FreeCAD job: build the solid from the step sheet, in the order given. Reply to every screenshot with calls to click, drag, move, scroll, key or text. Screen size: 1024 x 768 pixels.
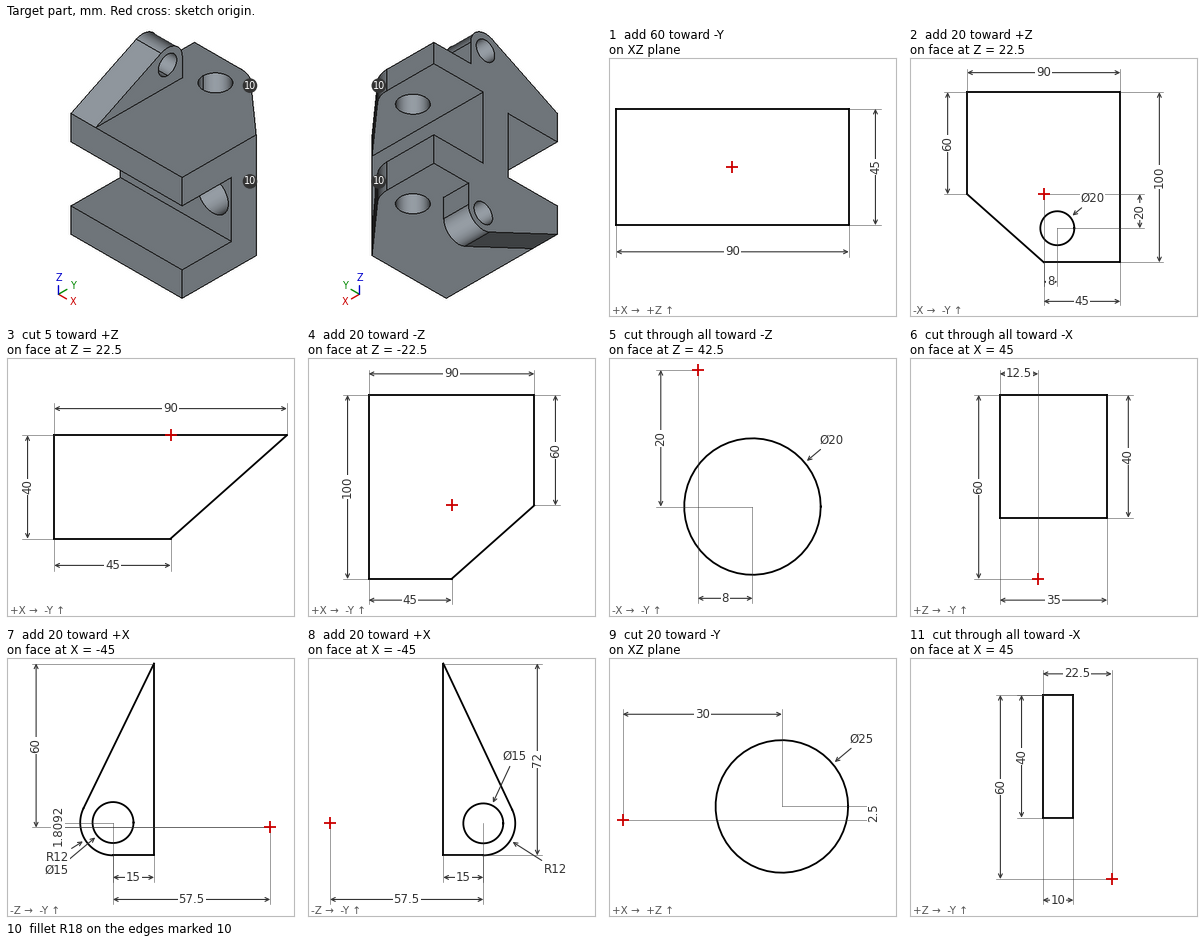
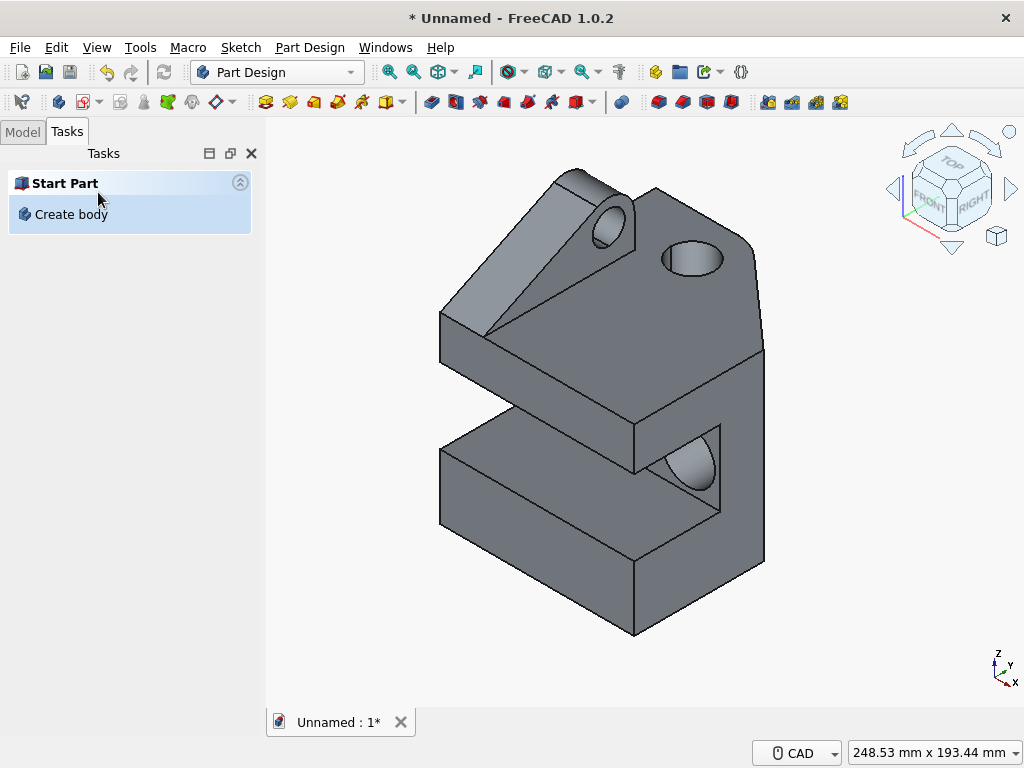
click(736, 531)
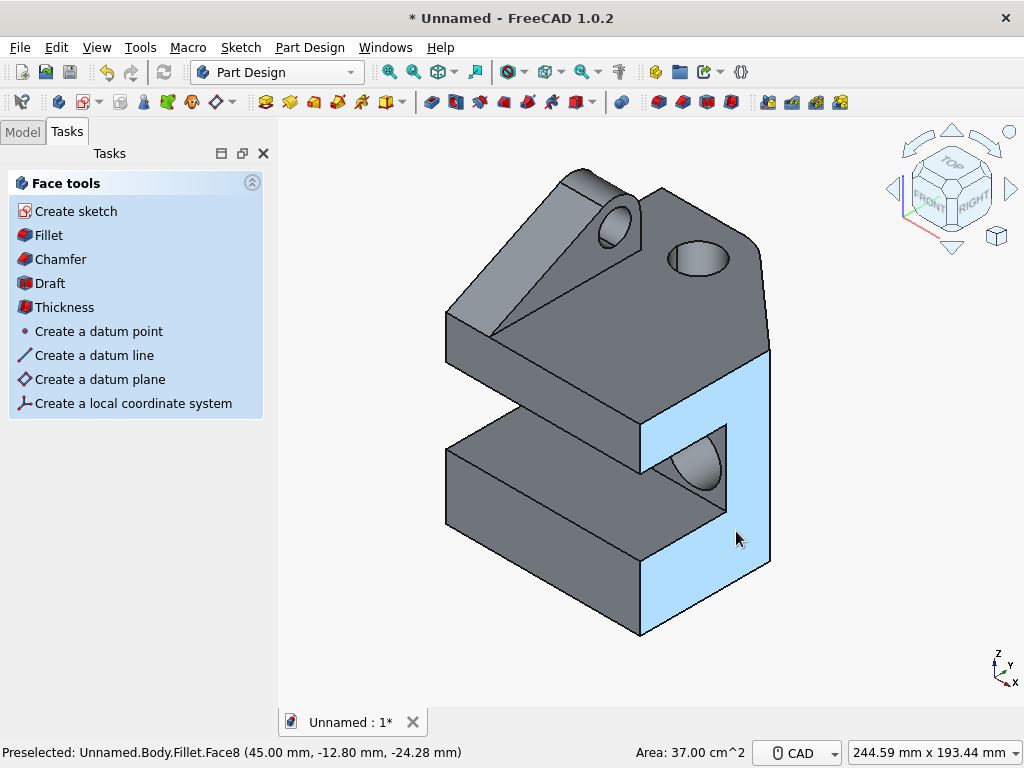
click(84, 102)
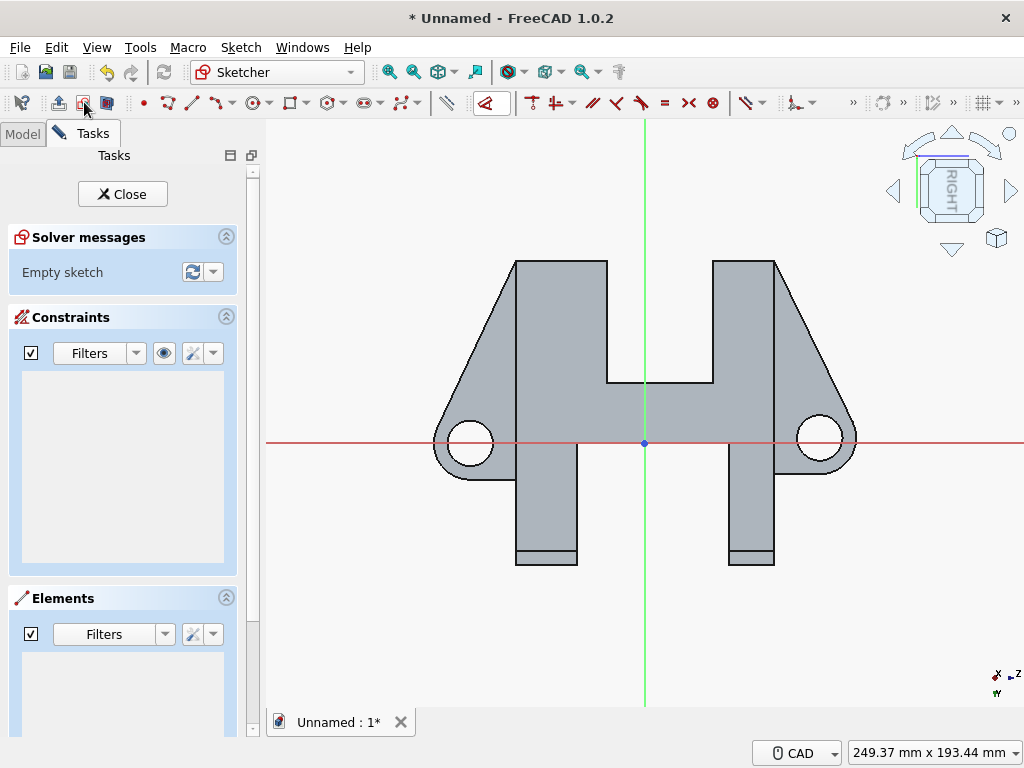
scroll(639, 303, up, 4)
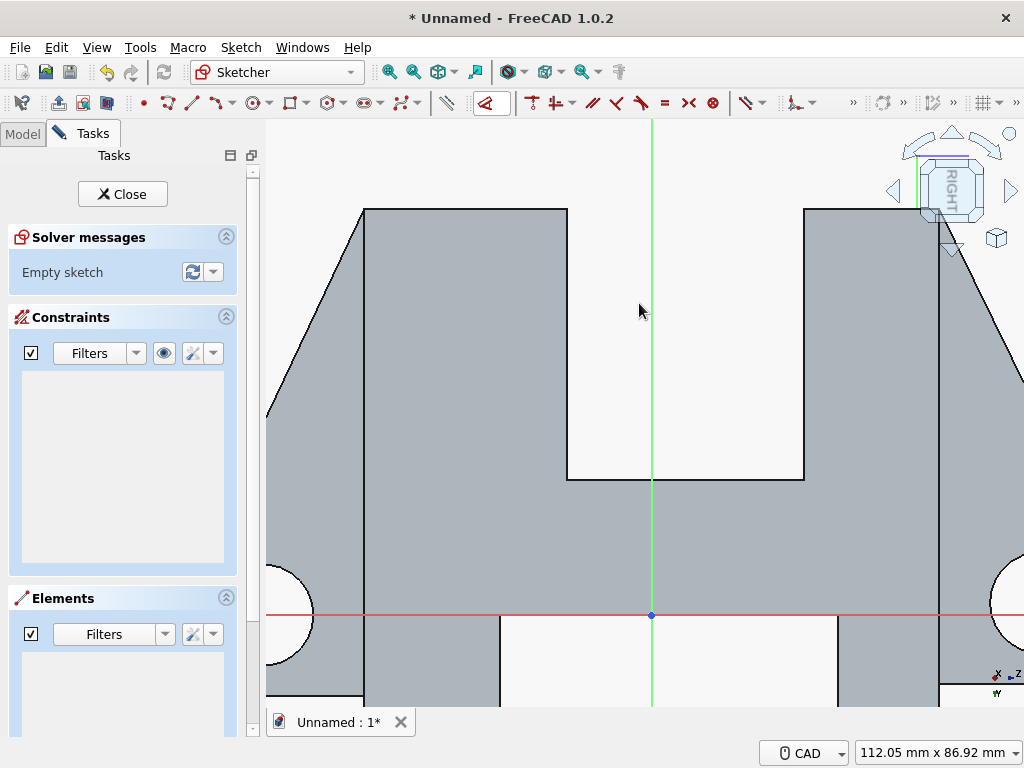
key(g)
key(r)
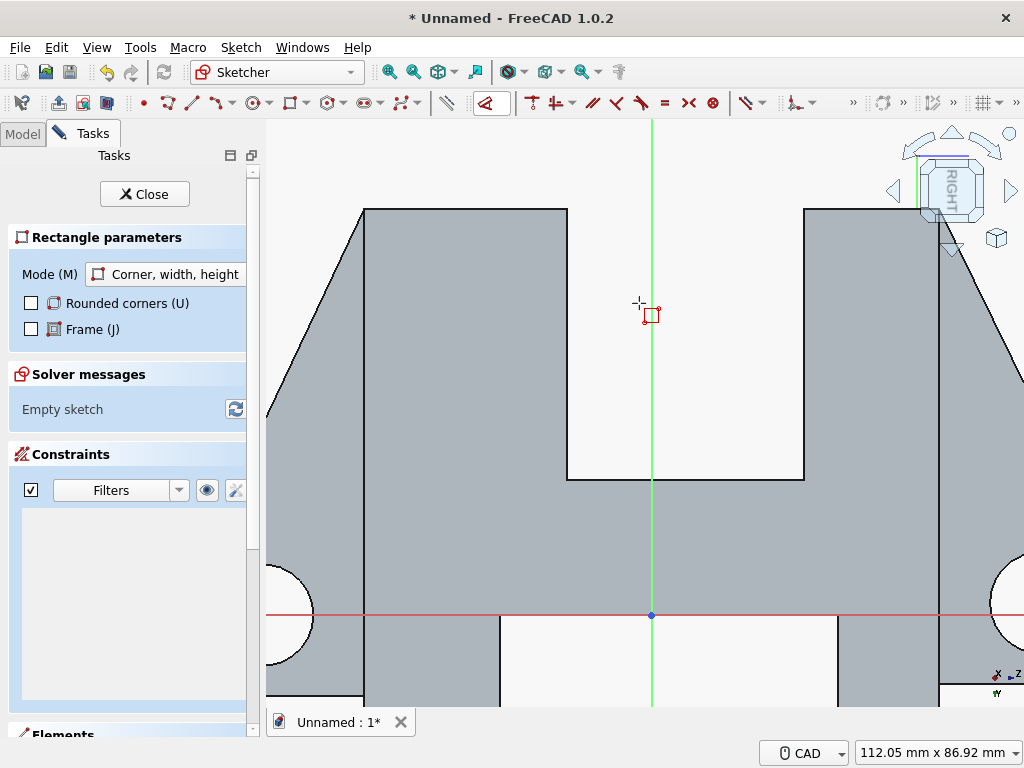
click(500, 209)
move(567, 480)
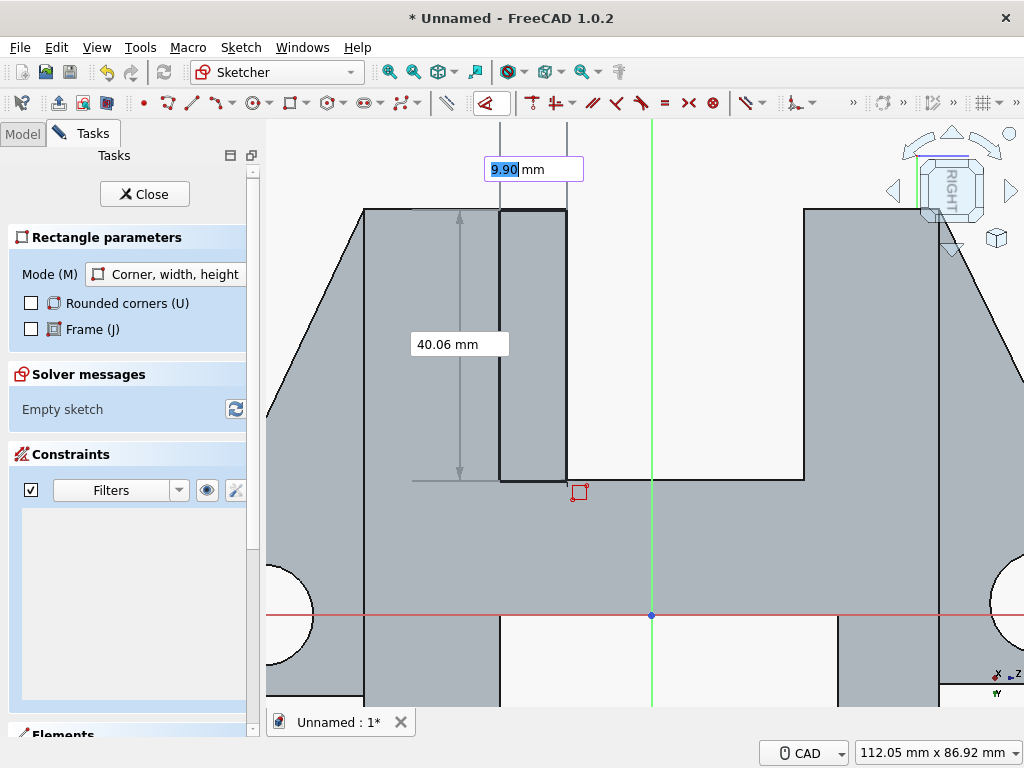
text(10)
key(Tab)
text(40)
key(Return)
key(Escape)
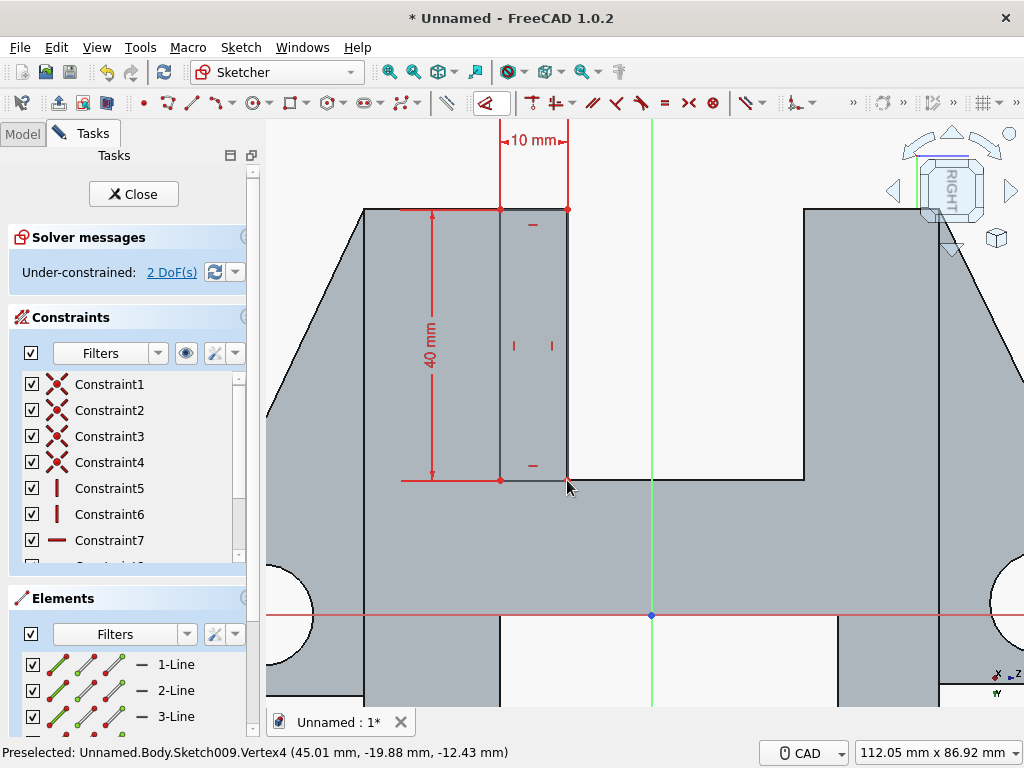
click(500, 210)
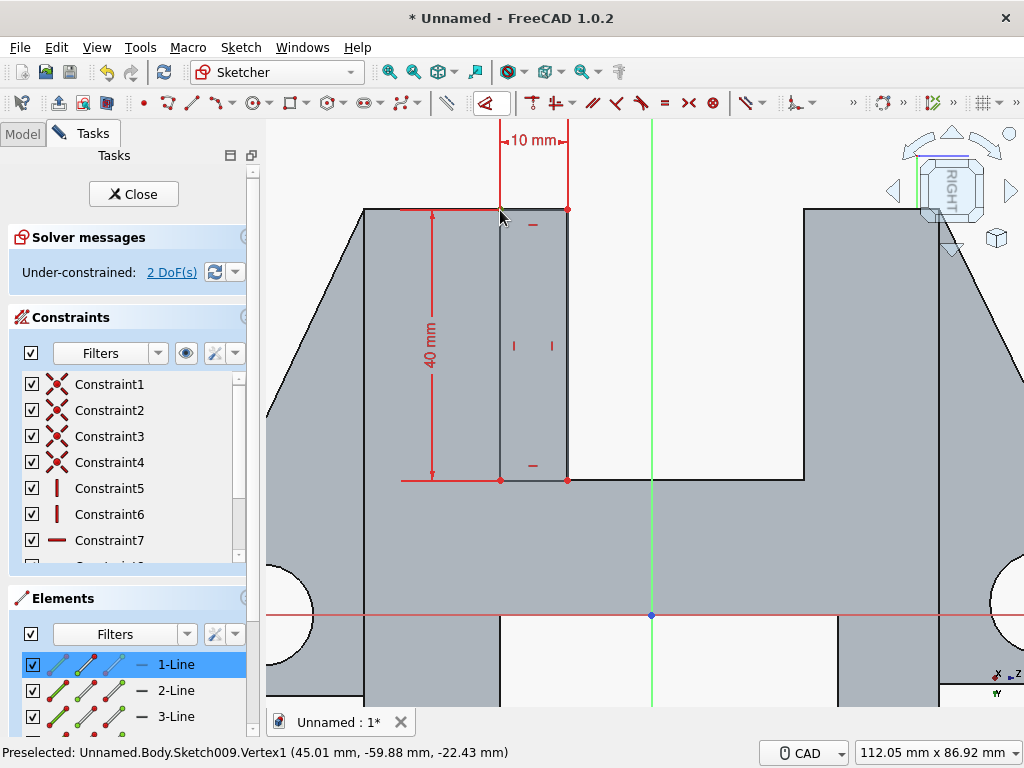
key(i)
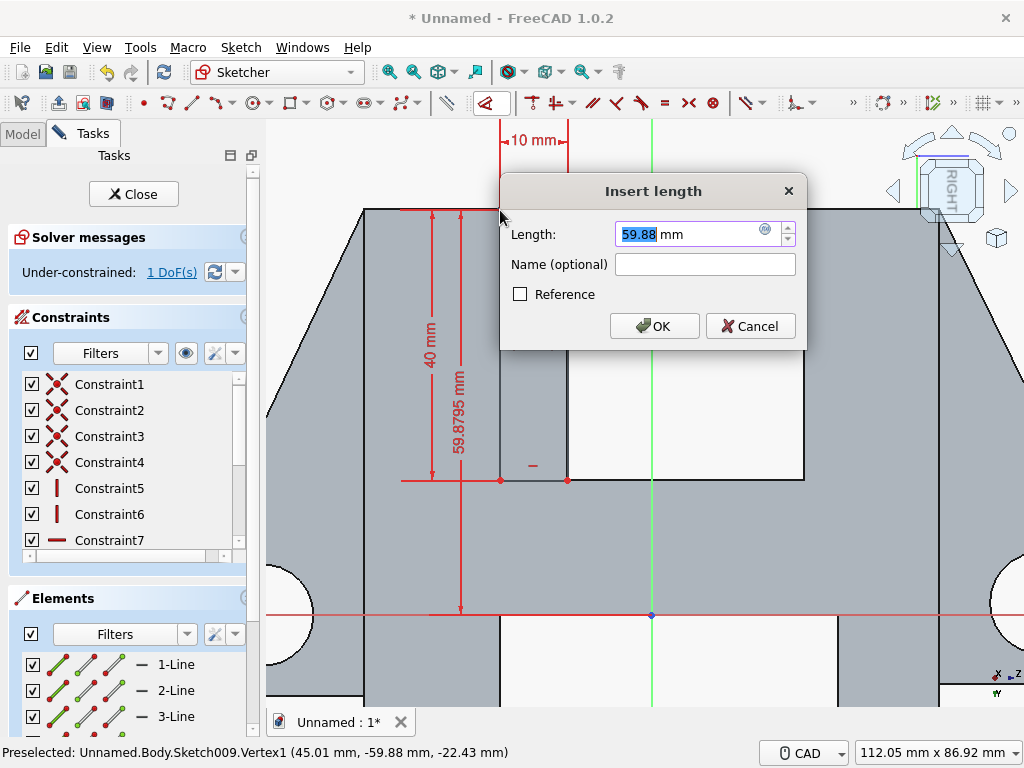
text(60)
key(Return)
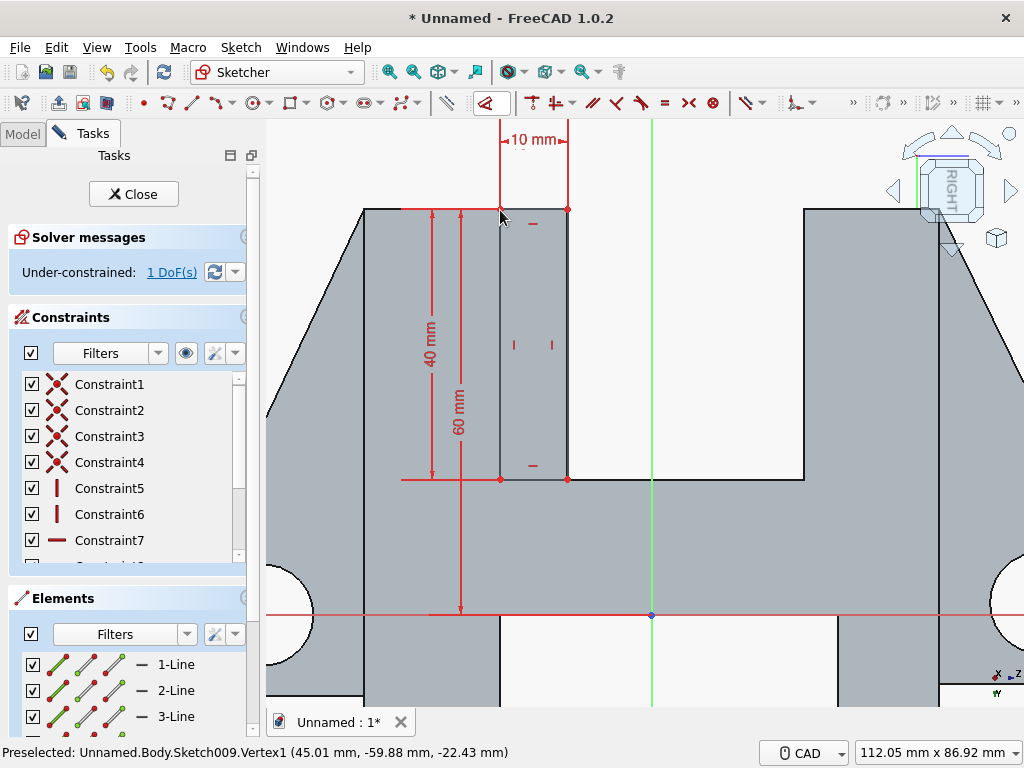
click(500, 209)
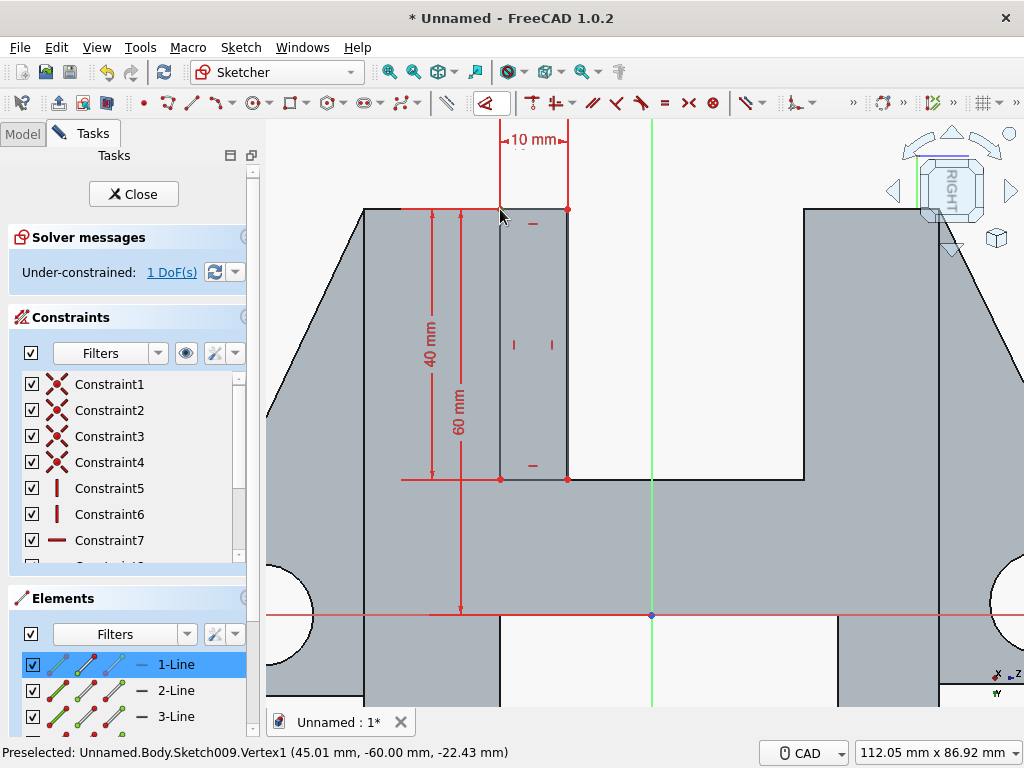
click(504, 104)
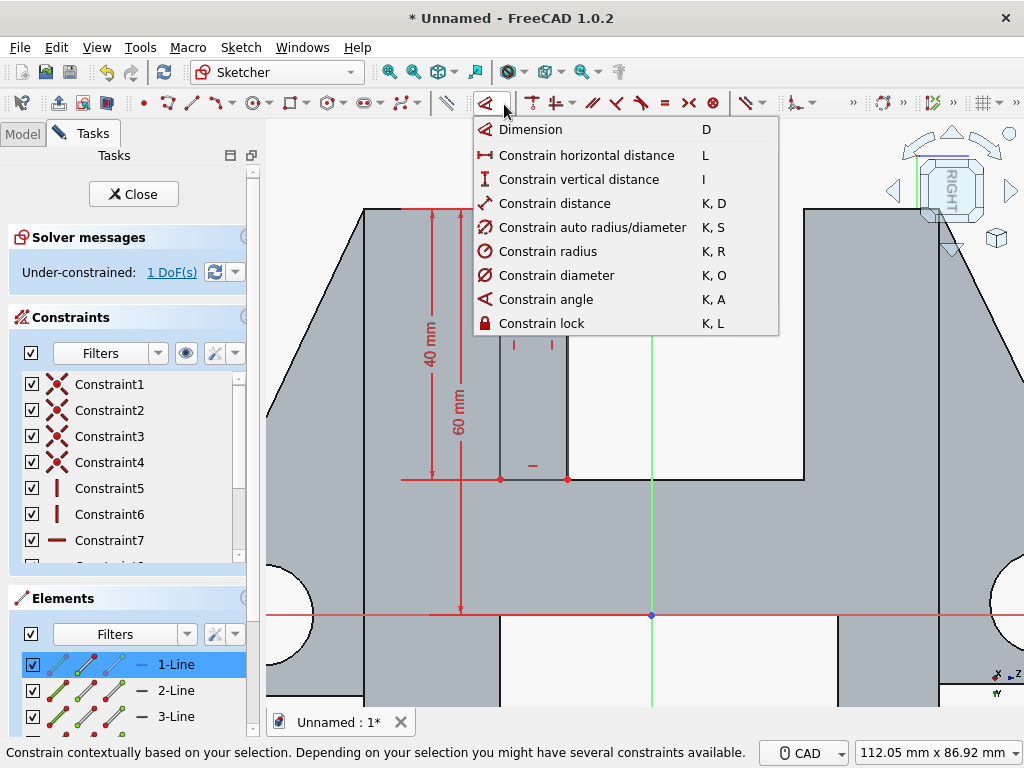
click(626, 155)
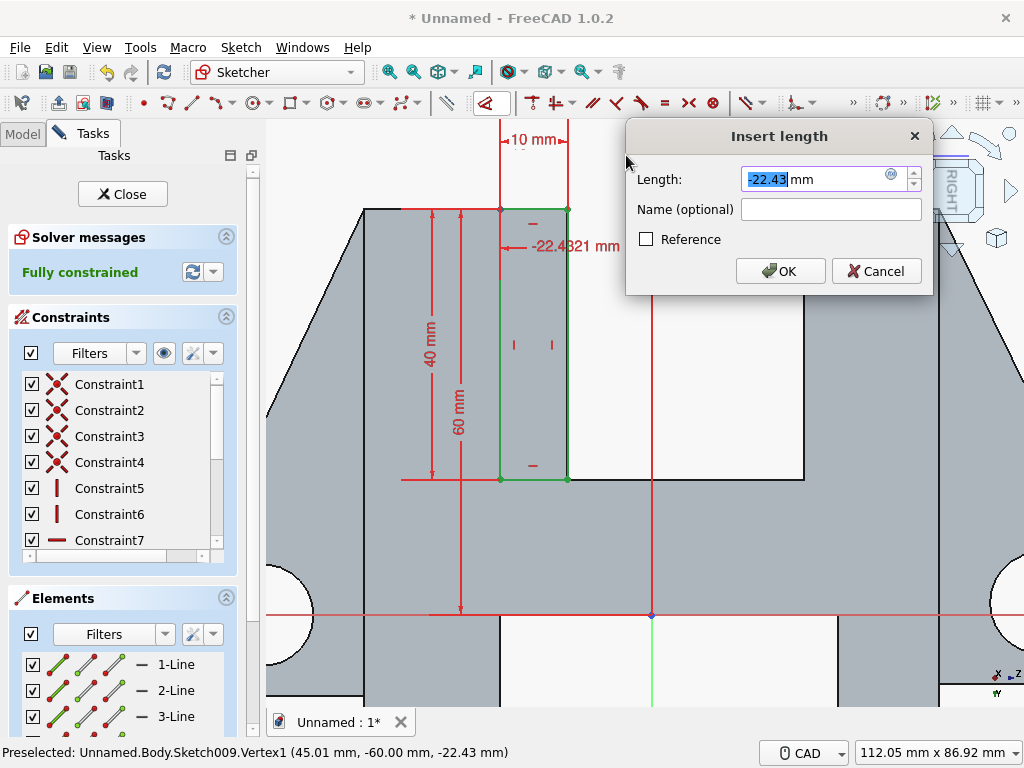
text(-22.5)
key(Return)